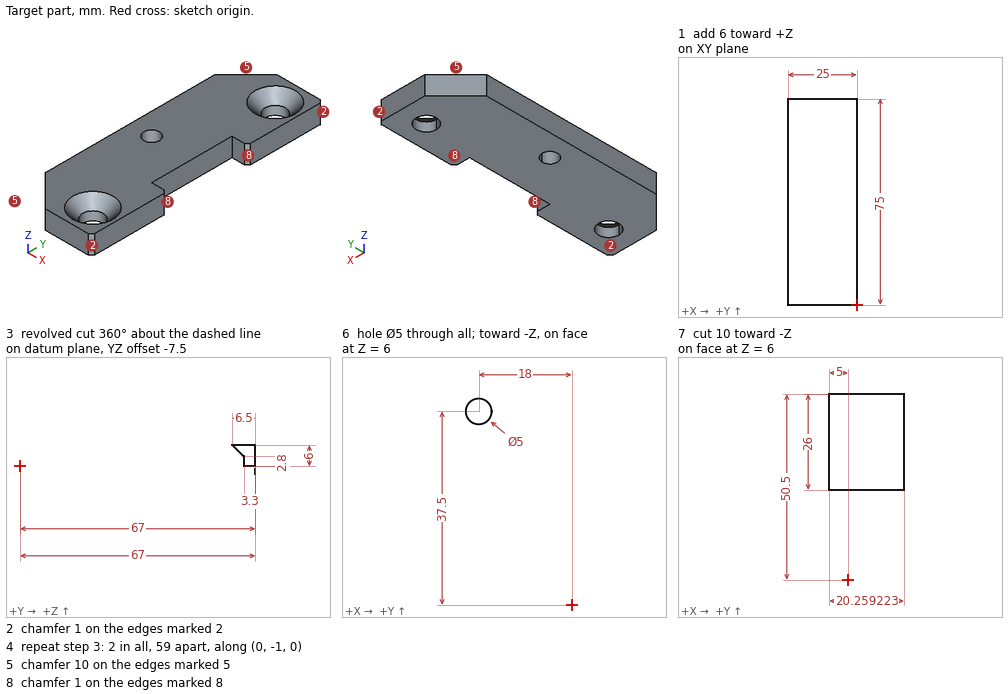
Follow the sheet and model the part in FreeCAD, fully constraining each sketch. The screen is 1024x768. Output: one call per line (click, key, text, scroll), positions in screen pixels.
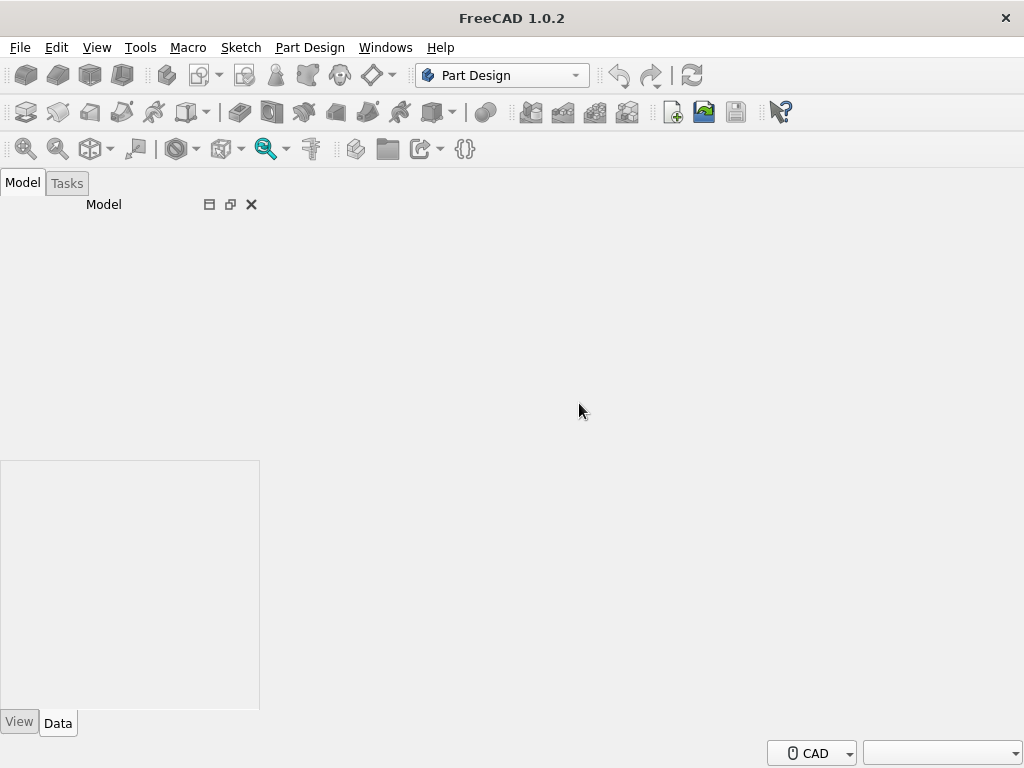
click(672, 112)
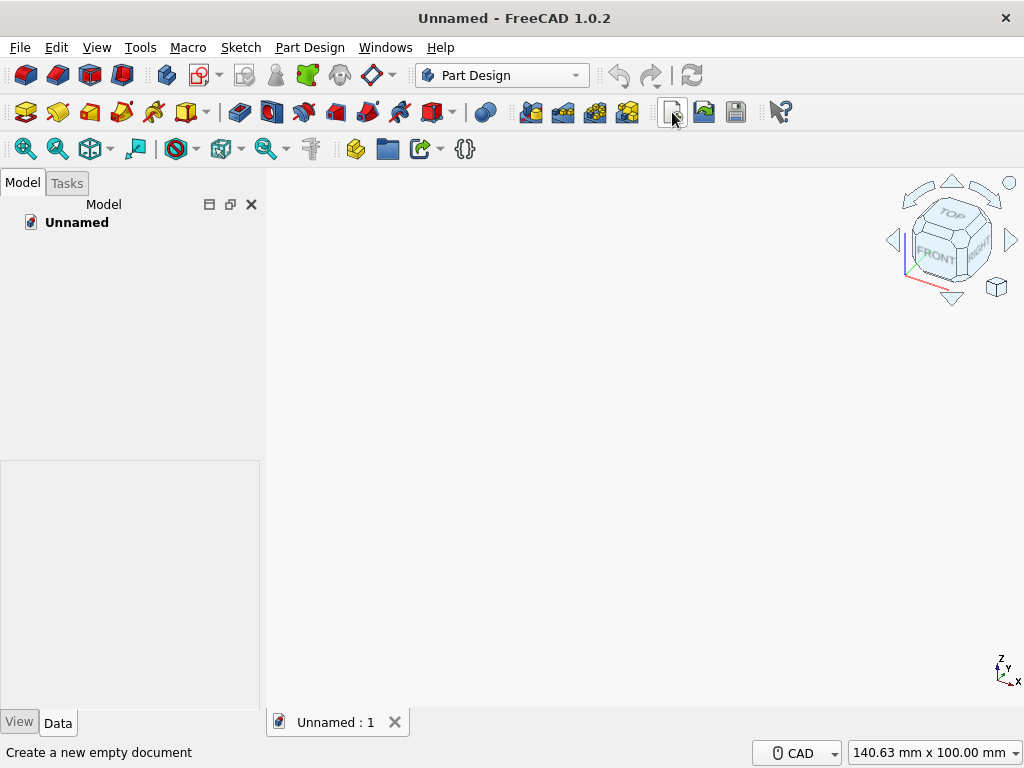
click(200, 76)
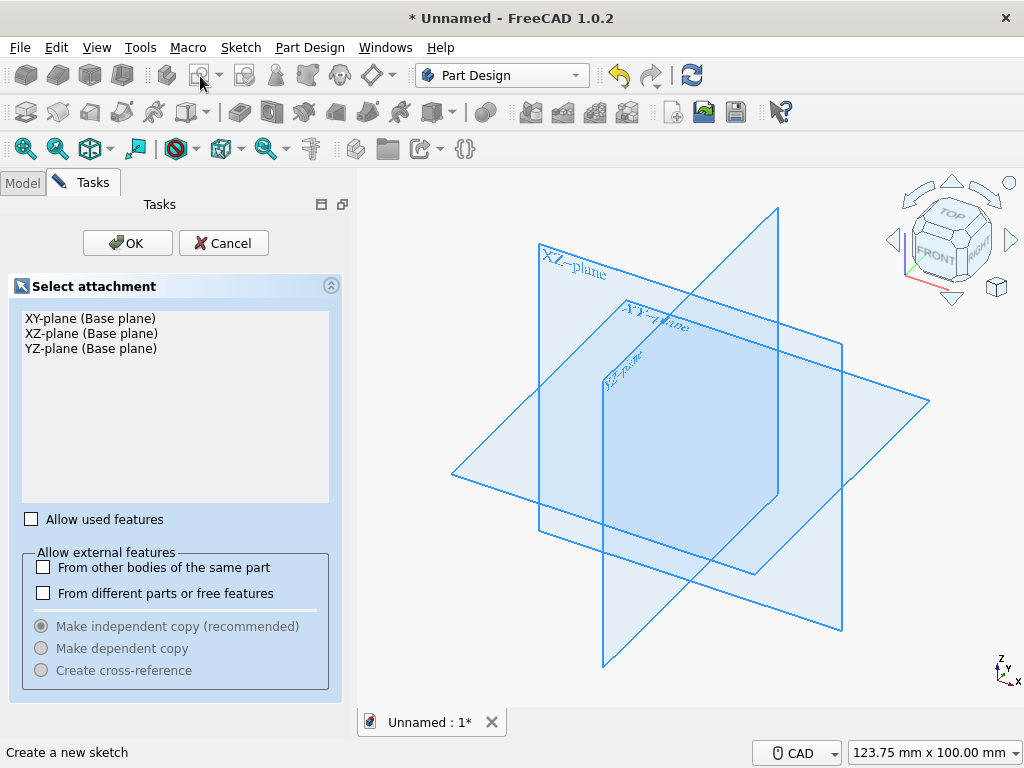
click(82, 318)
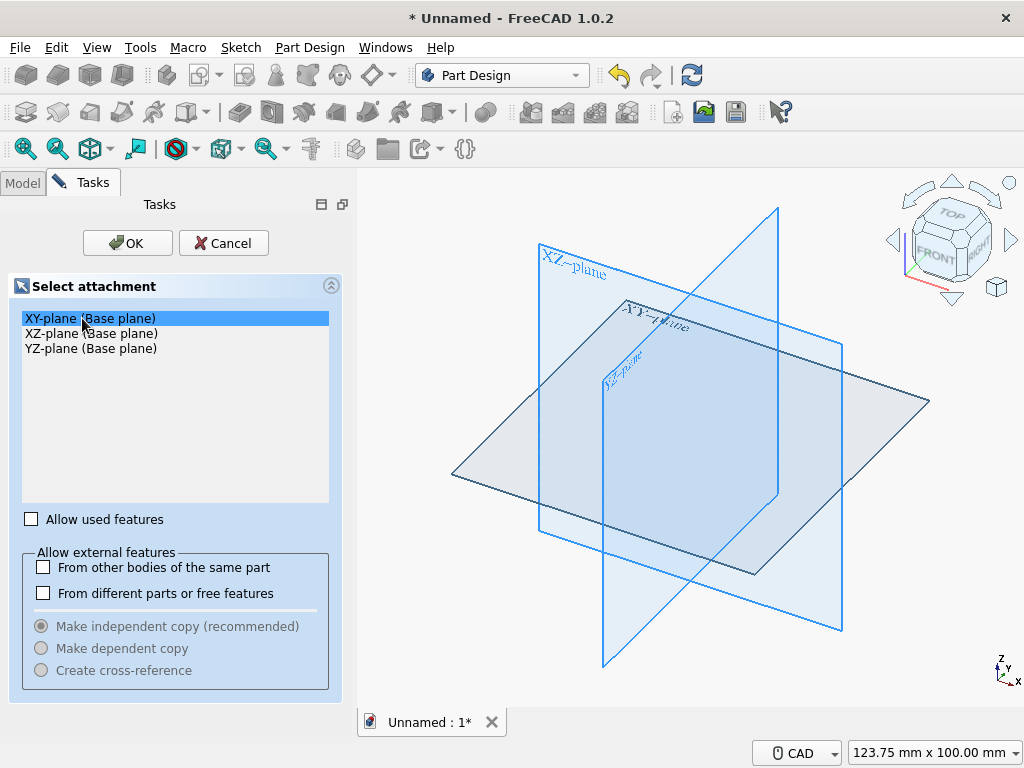
click(128, 243)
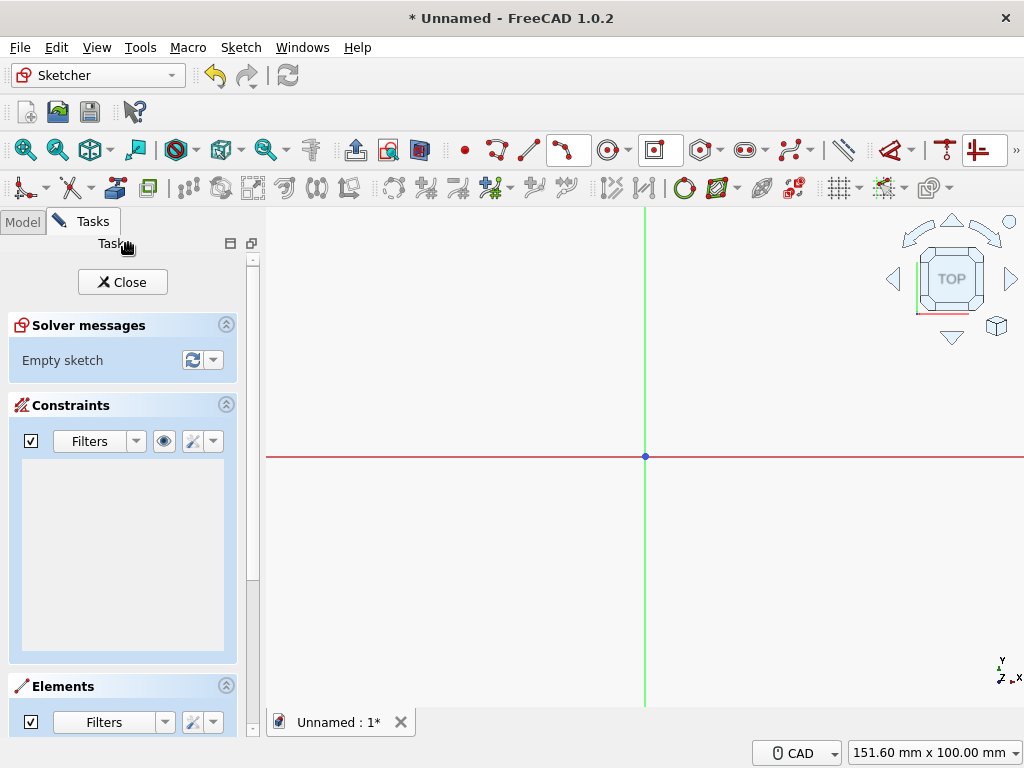
scroll(564, 679, down, 2)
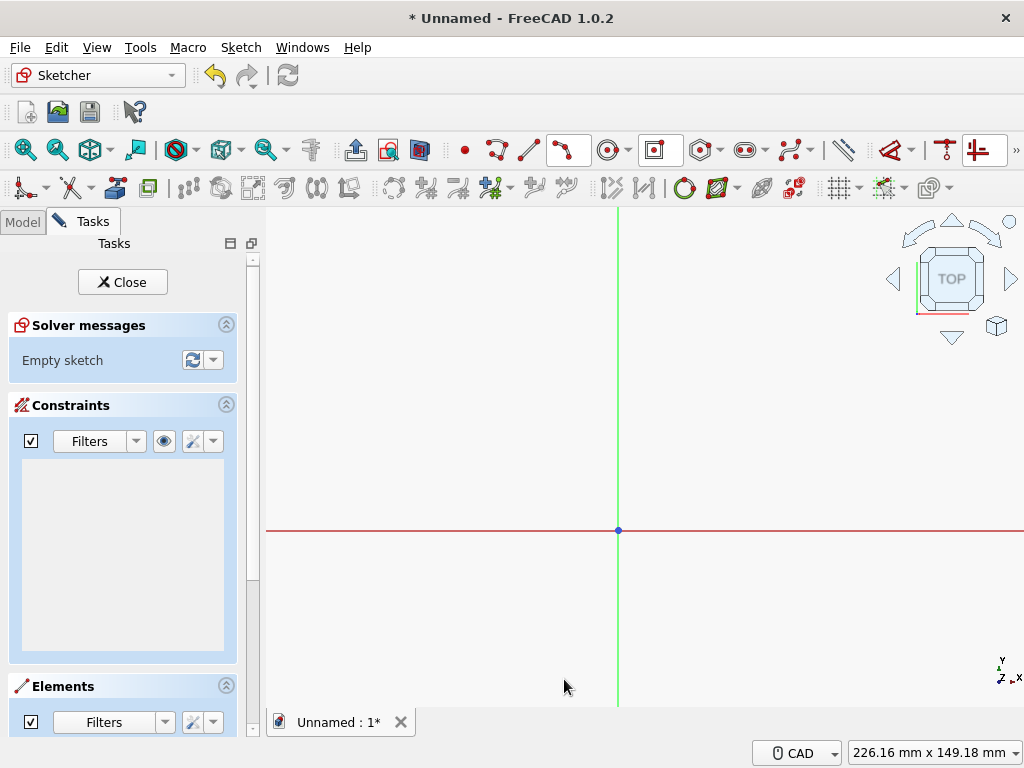
click(678, 150)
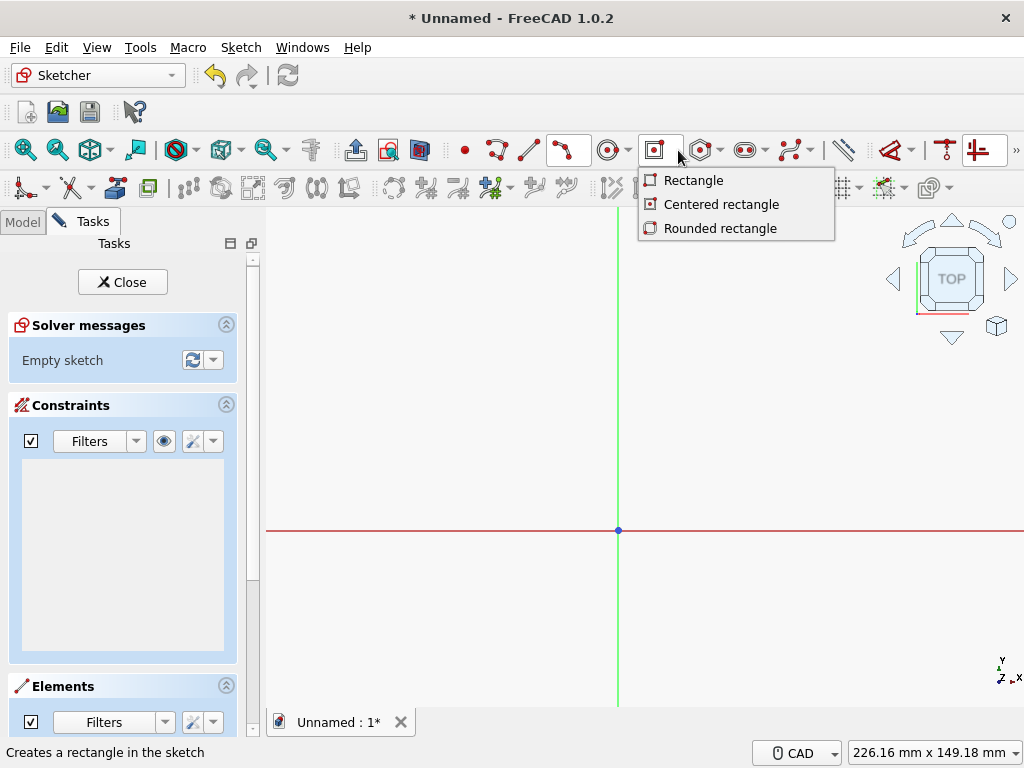
click(736, 180)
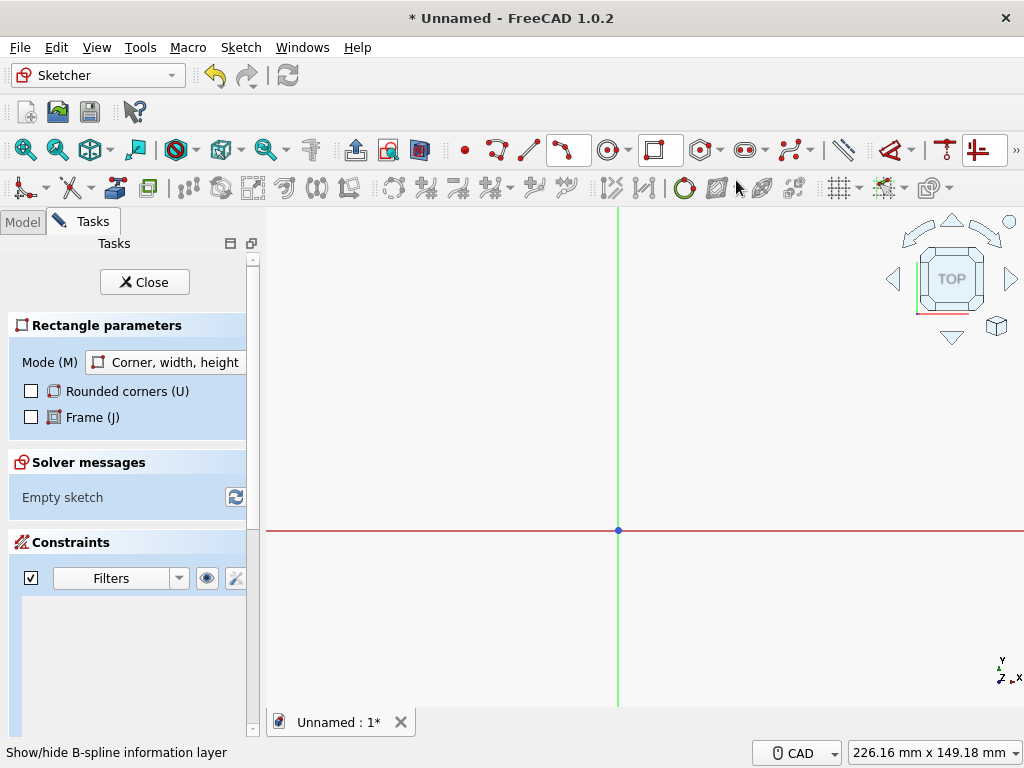
click(618, 531)
click(535, 279)
key(Escape)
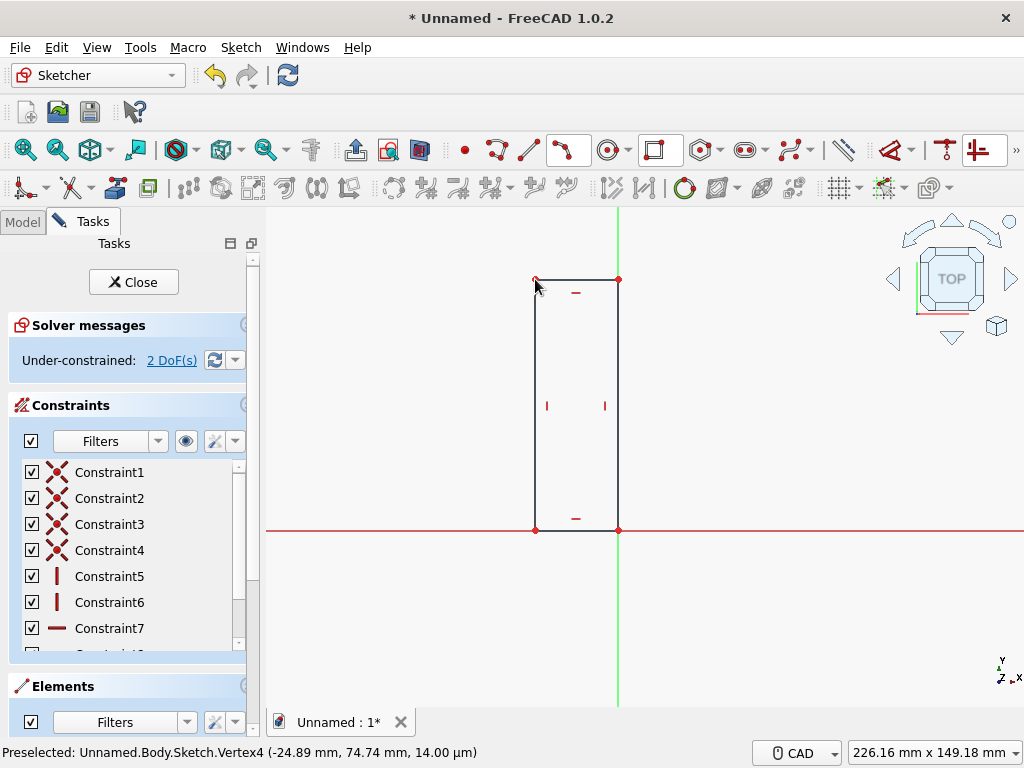
click(890, 150)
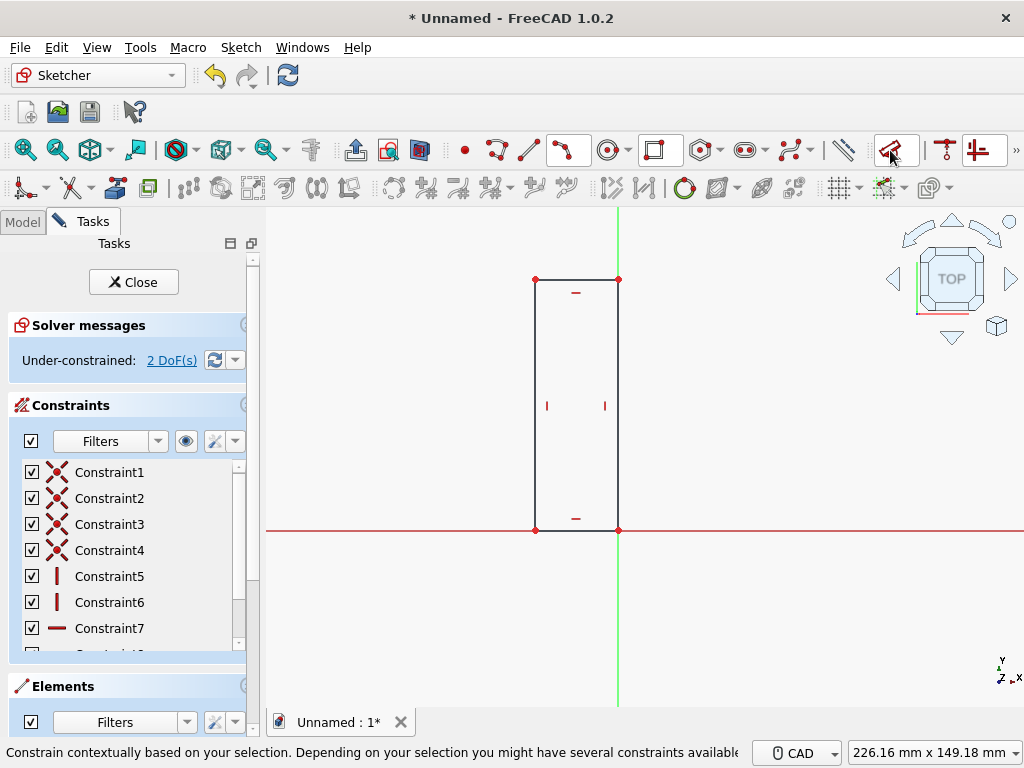
click(618, 455)
click(652, 405)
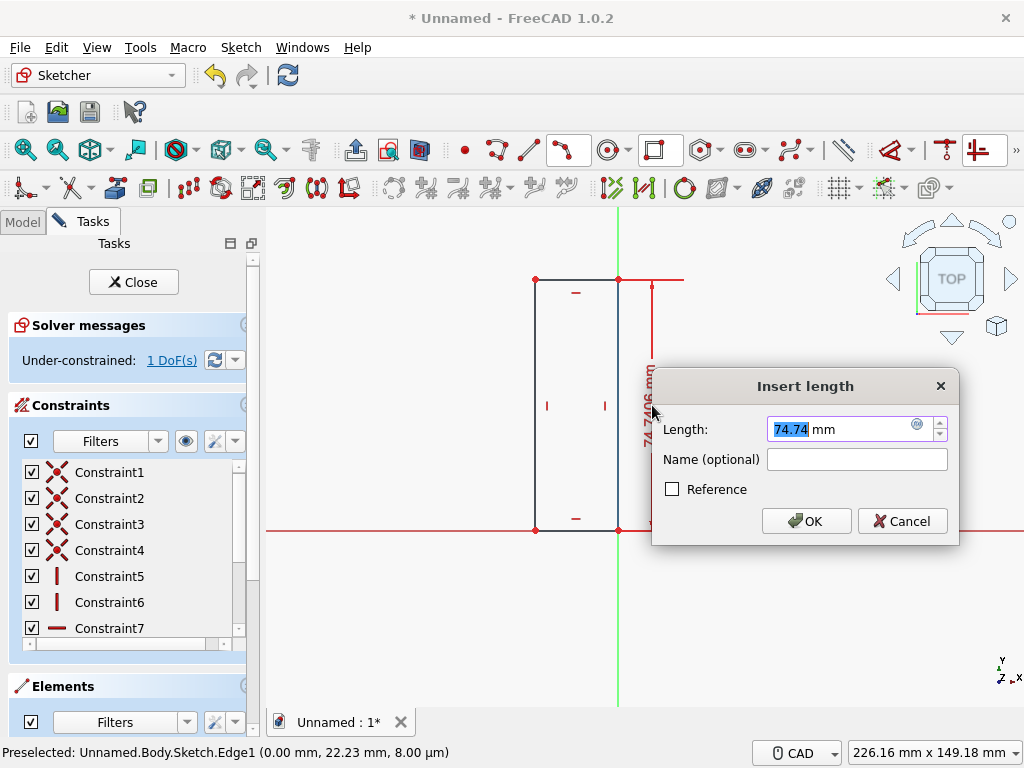
text(75)
key(Return)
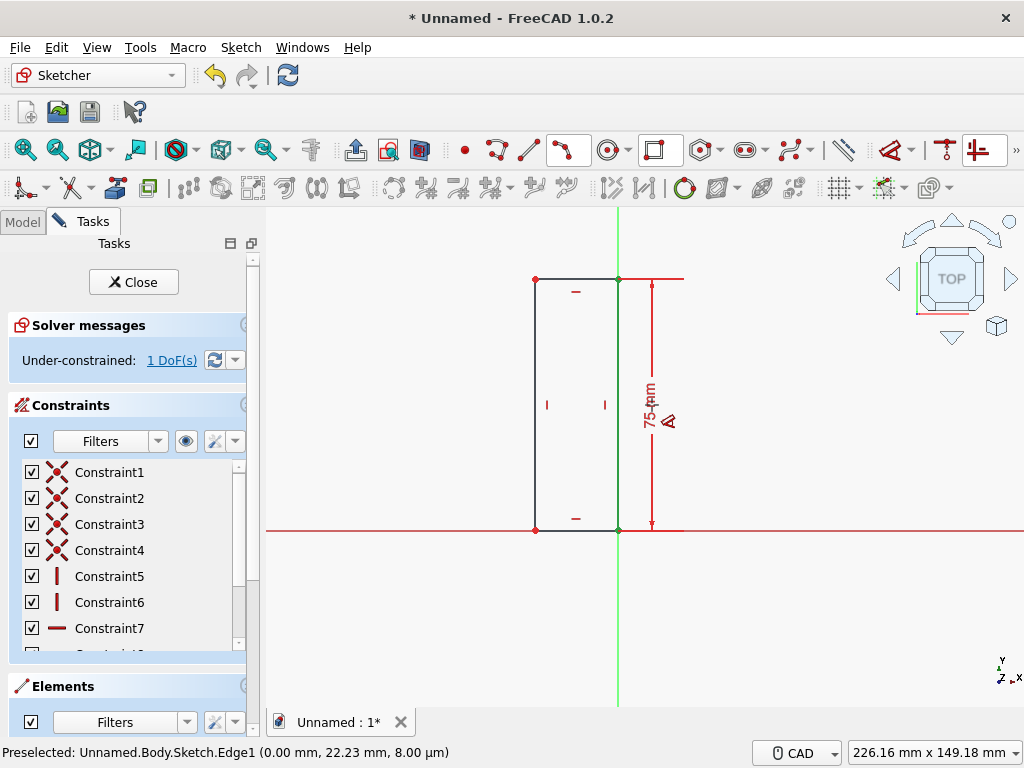
click(593, 279)
click(577, 245)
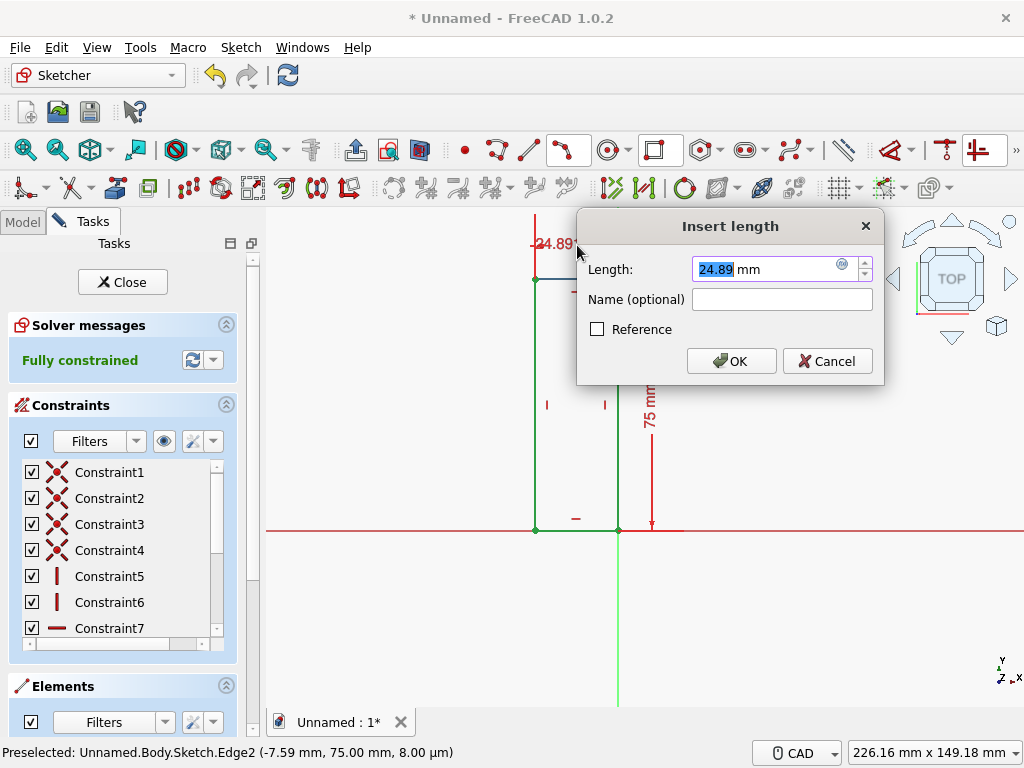
text(25)
key(Return)
key(Escape)